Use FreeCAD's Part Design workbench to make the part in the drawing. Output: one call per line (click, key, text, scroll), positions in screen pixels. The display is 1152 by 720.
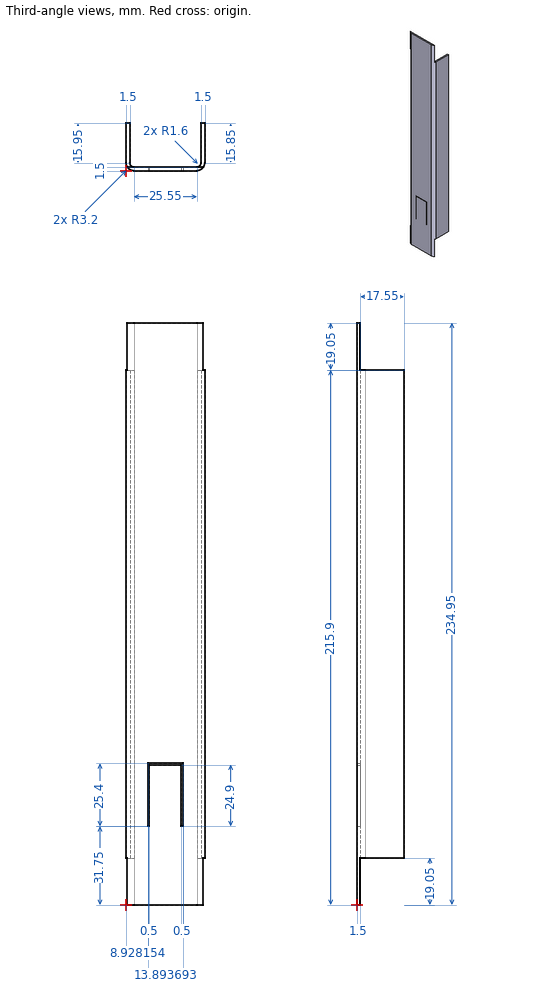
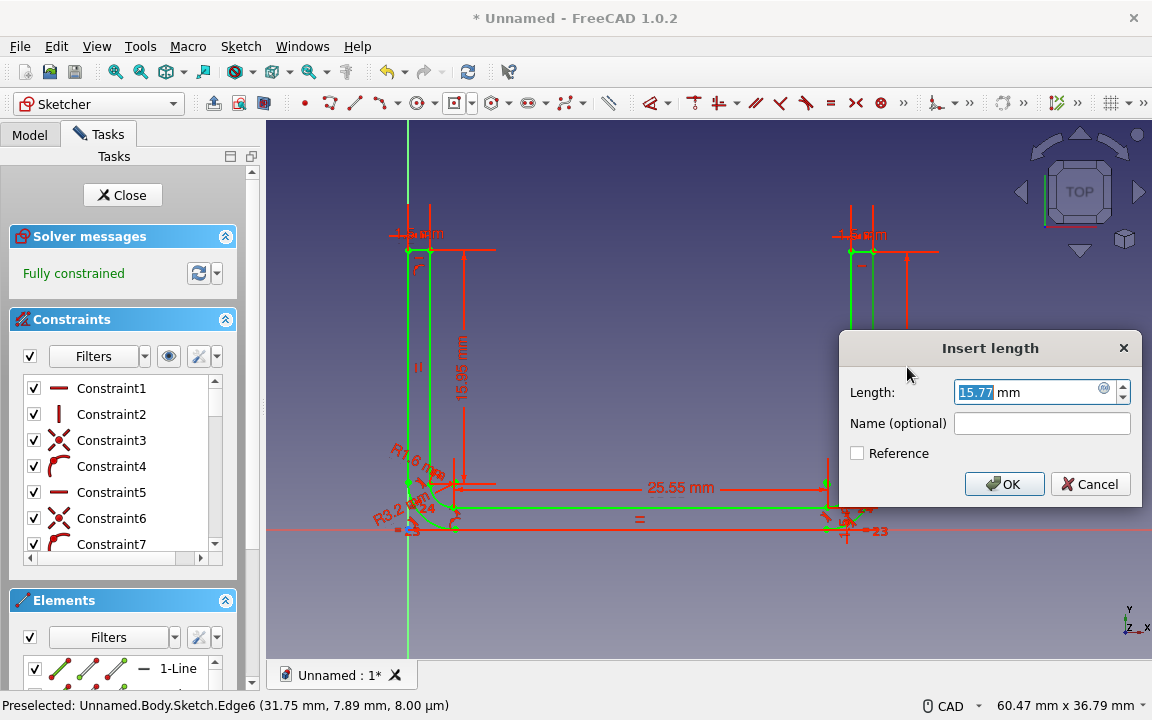
text(15.85)
key(Return)
key(Escape)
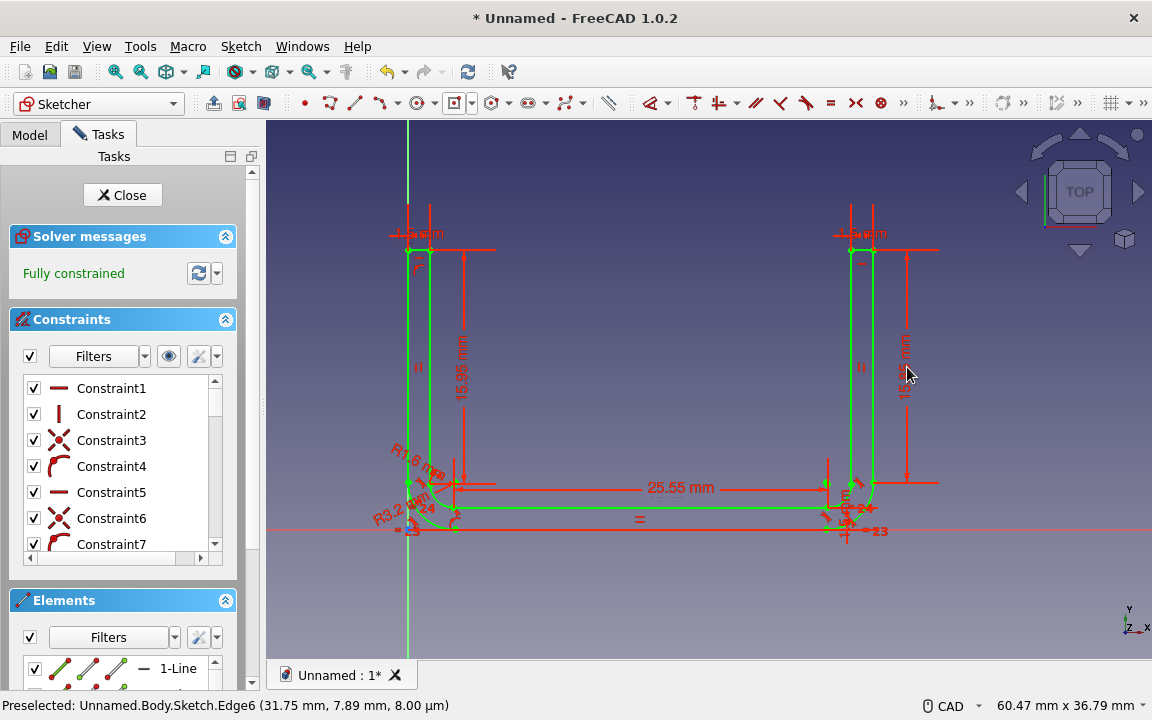
click(123, 195)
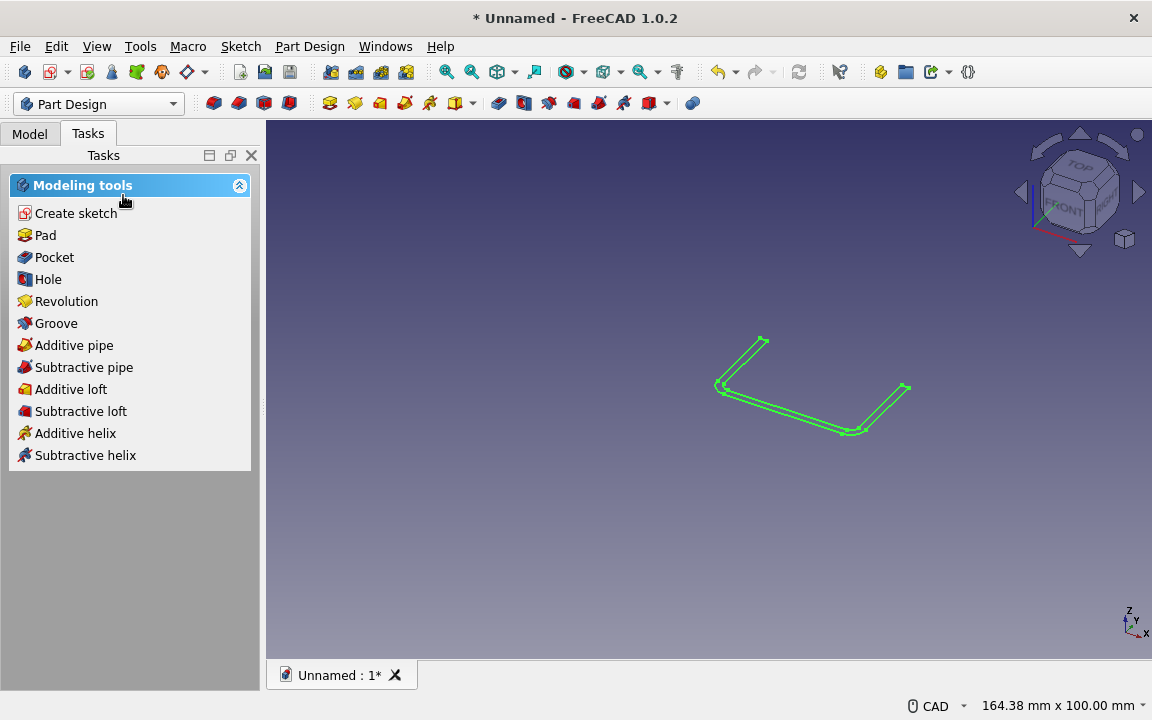
click(330, 104)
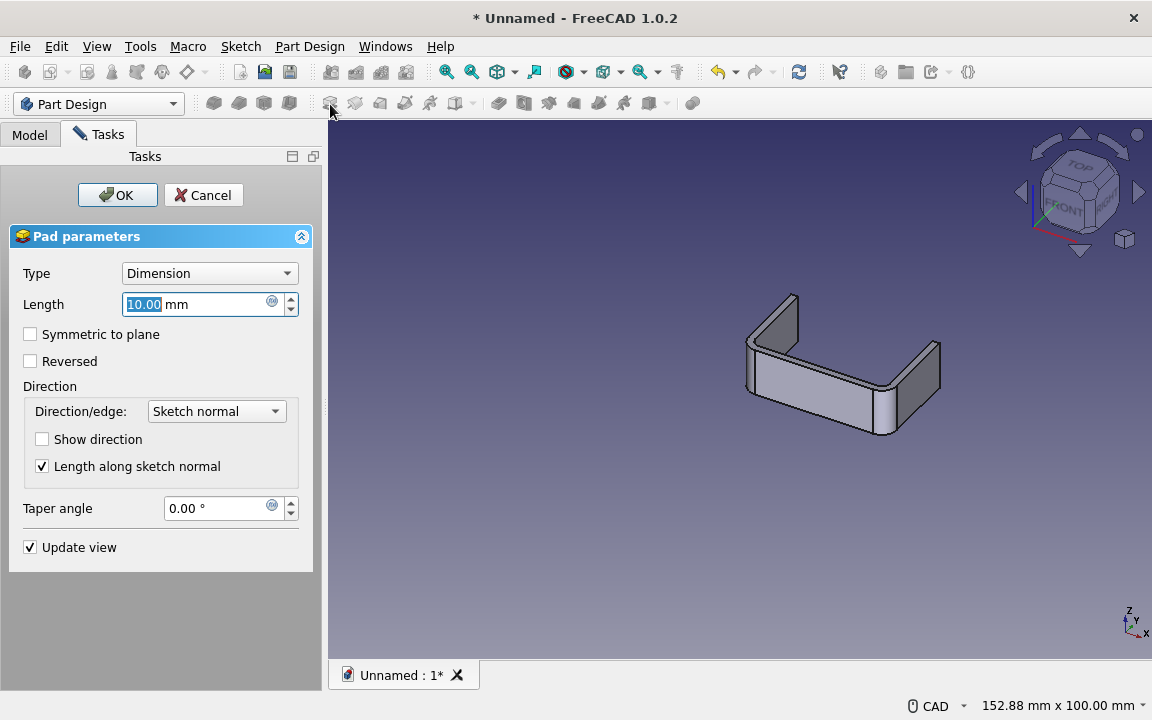
text(234.95)
key(Tab)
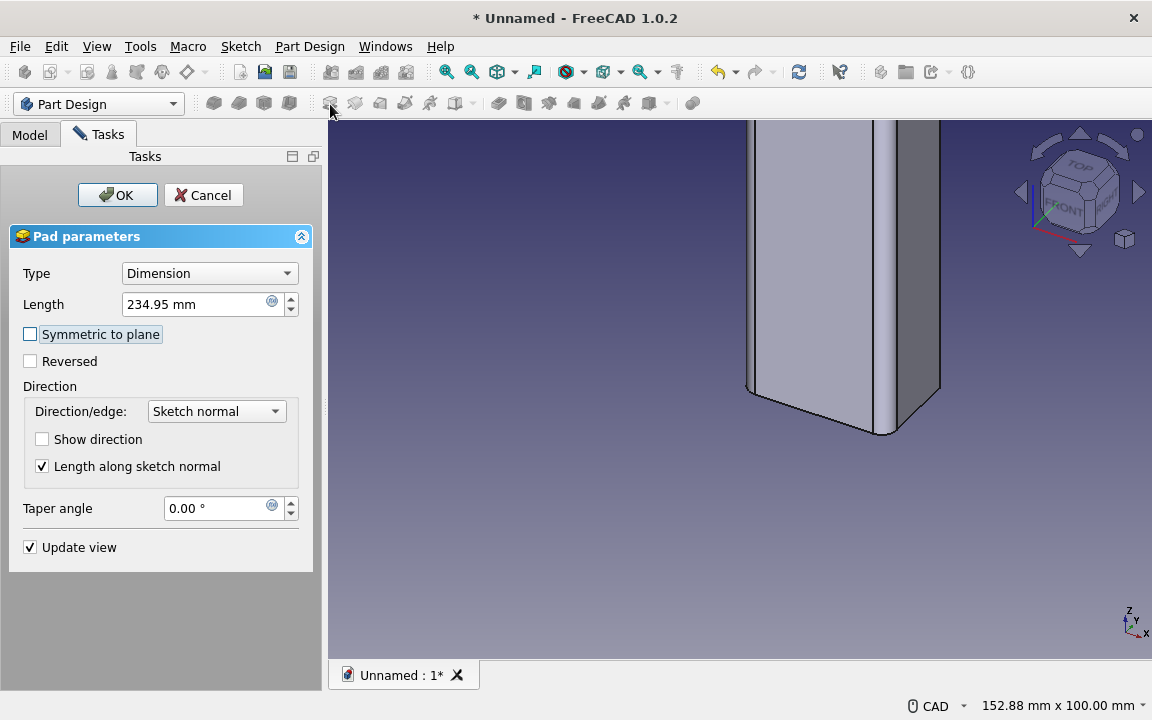
click(118, 195)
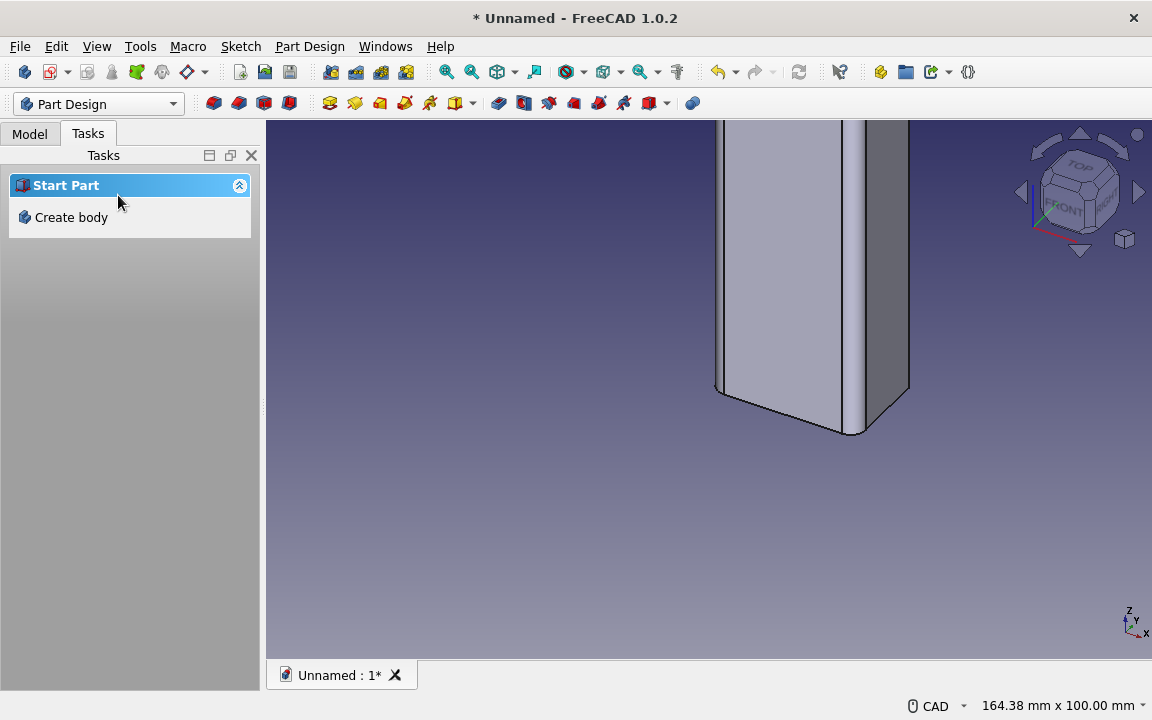
key(v)
key(f)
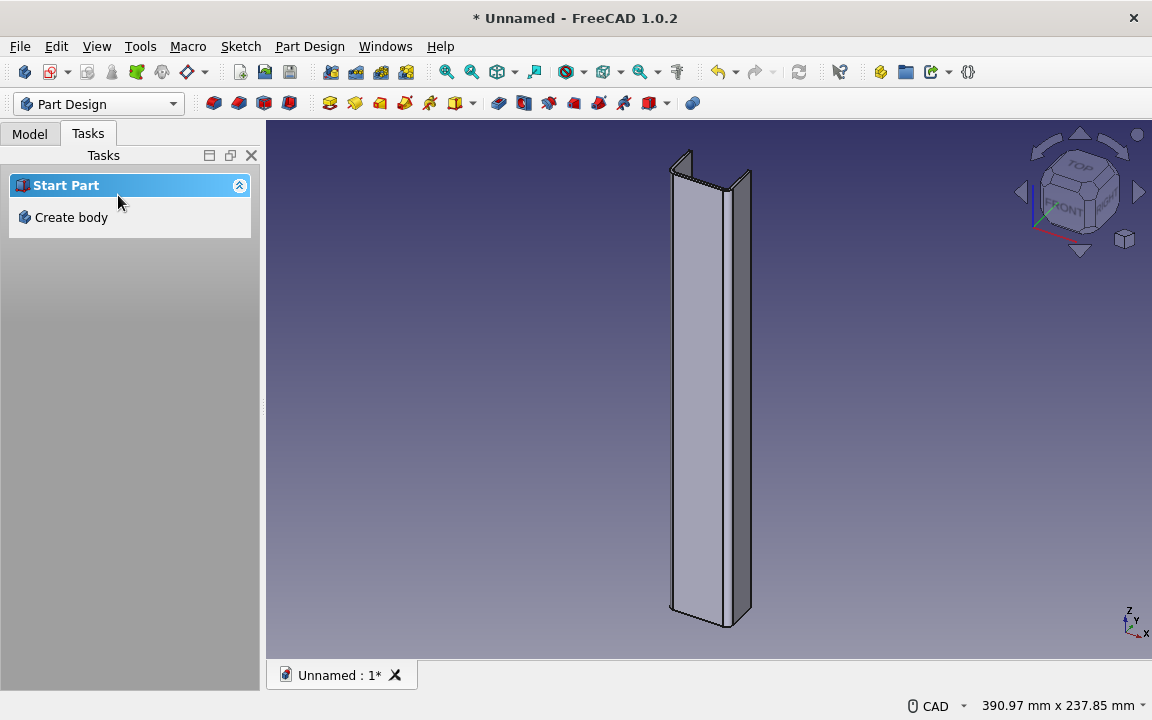
key(6)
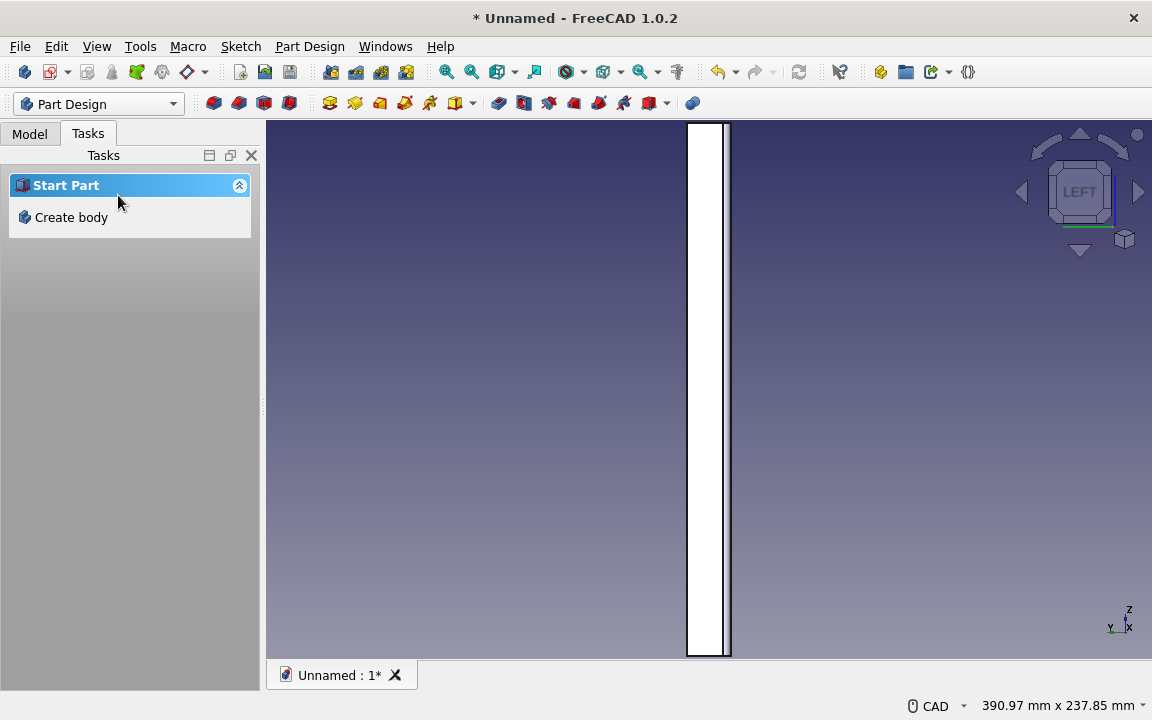
click(705, 160)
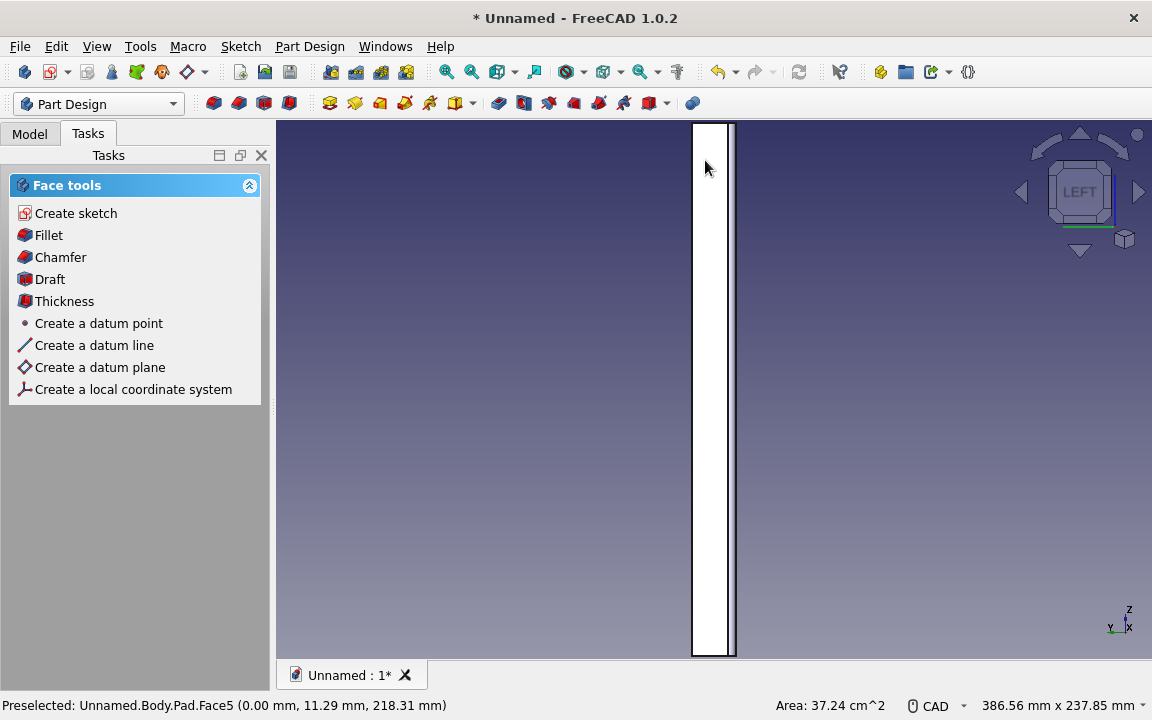
click(50, 72)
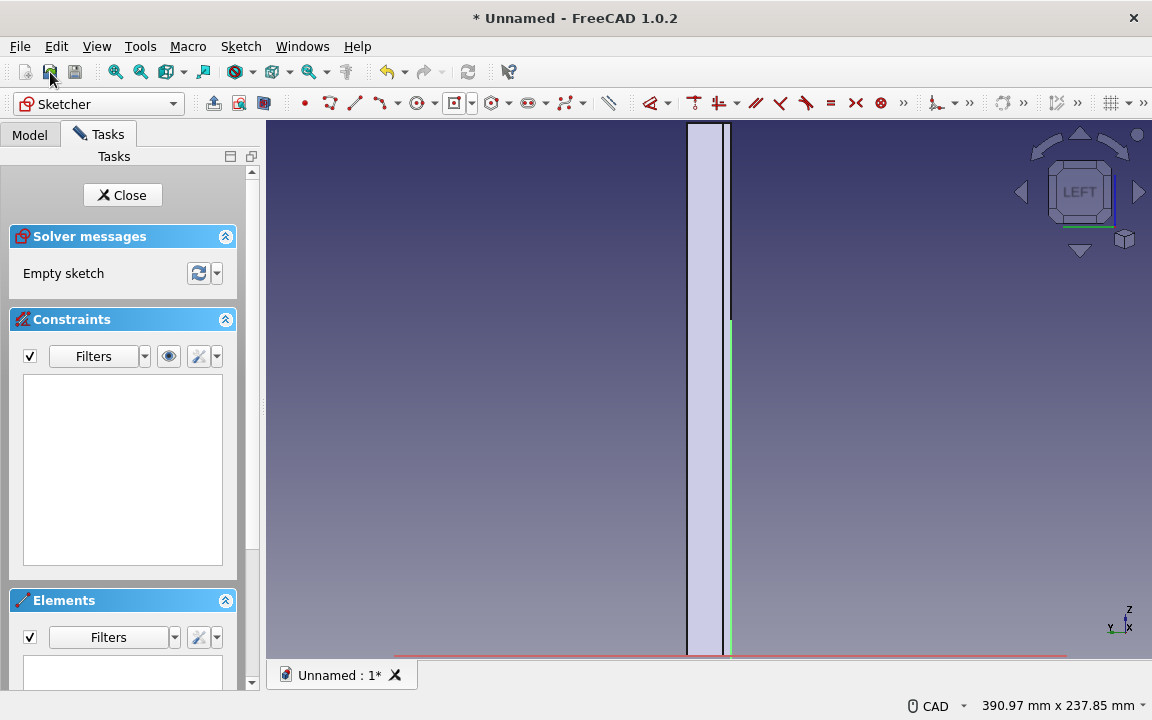
scroll(501, 390, down, 2)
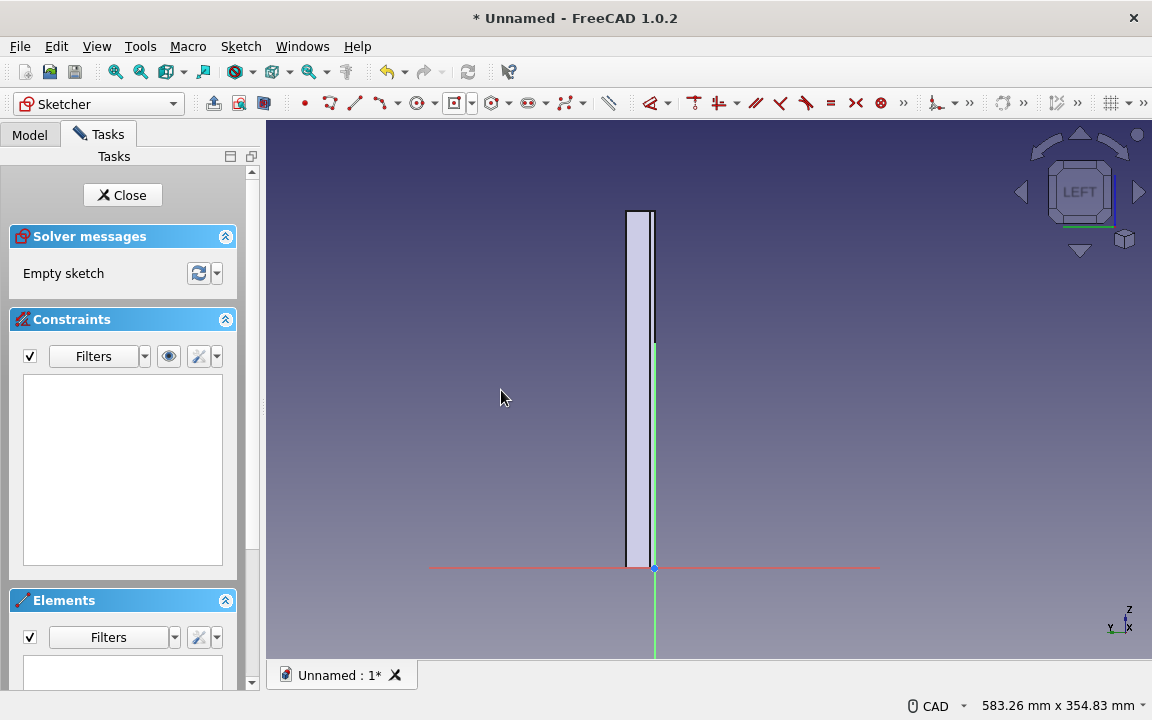
key(g)
key(r)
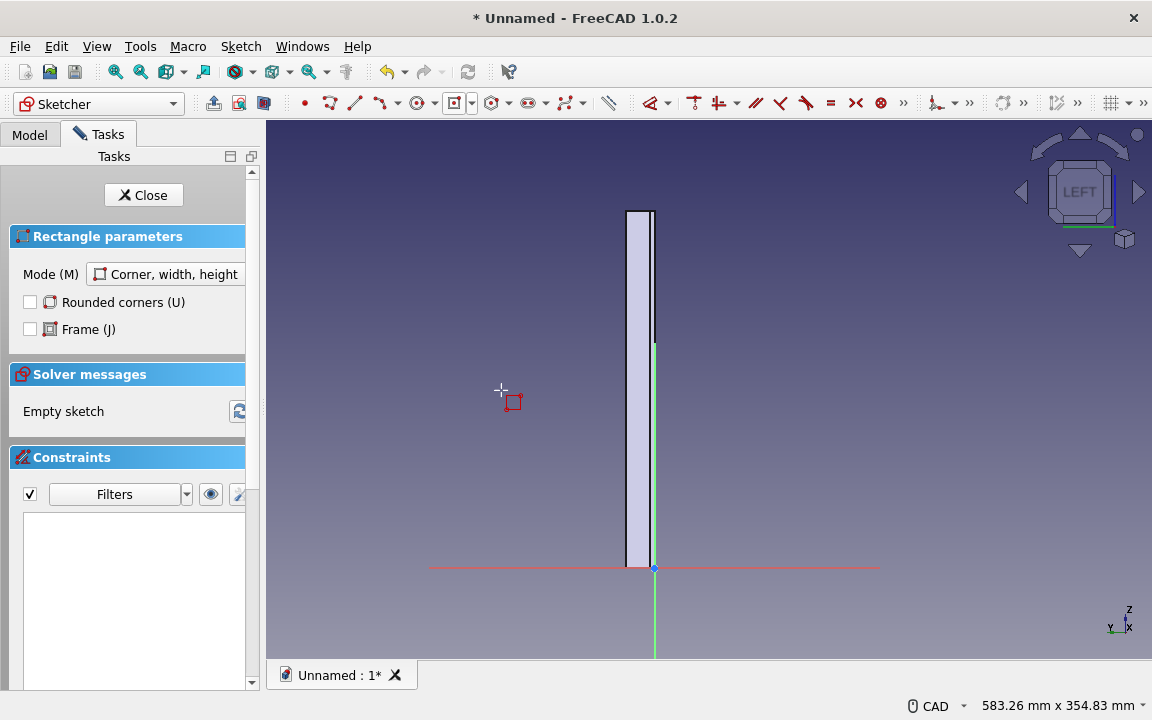
click(626, 539)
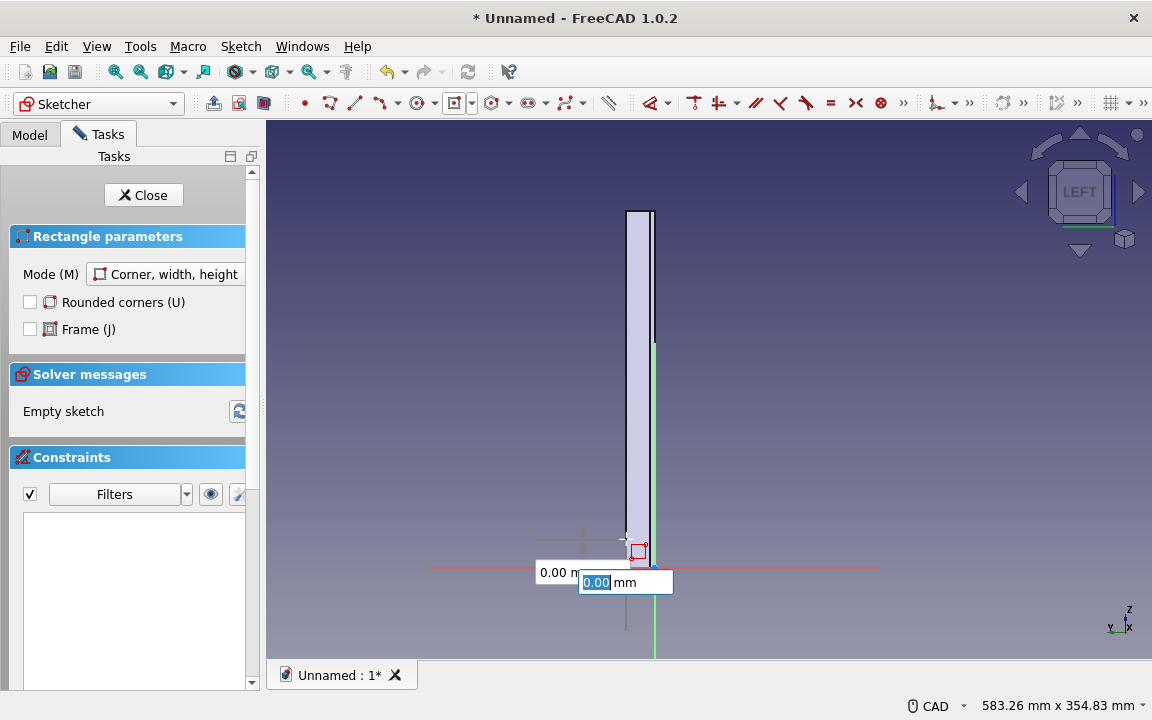
scroll(653, 568, up, 10)